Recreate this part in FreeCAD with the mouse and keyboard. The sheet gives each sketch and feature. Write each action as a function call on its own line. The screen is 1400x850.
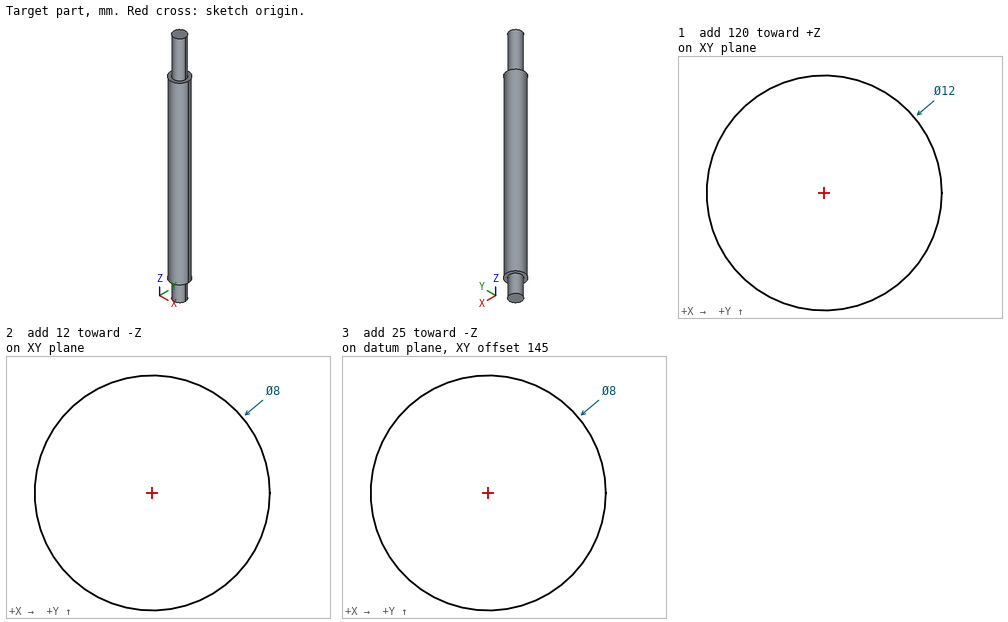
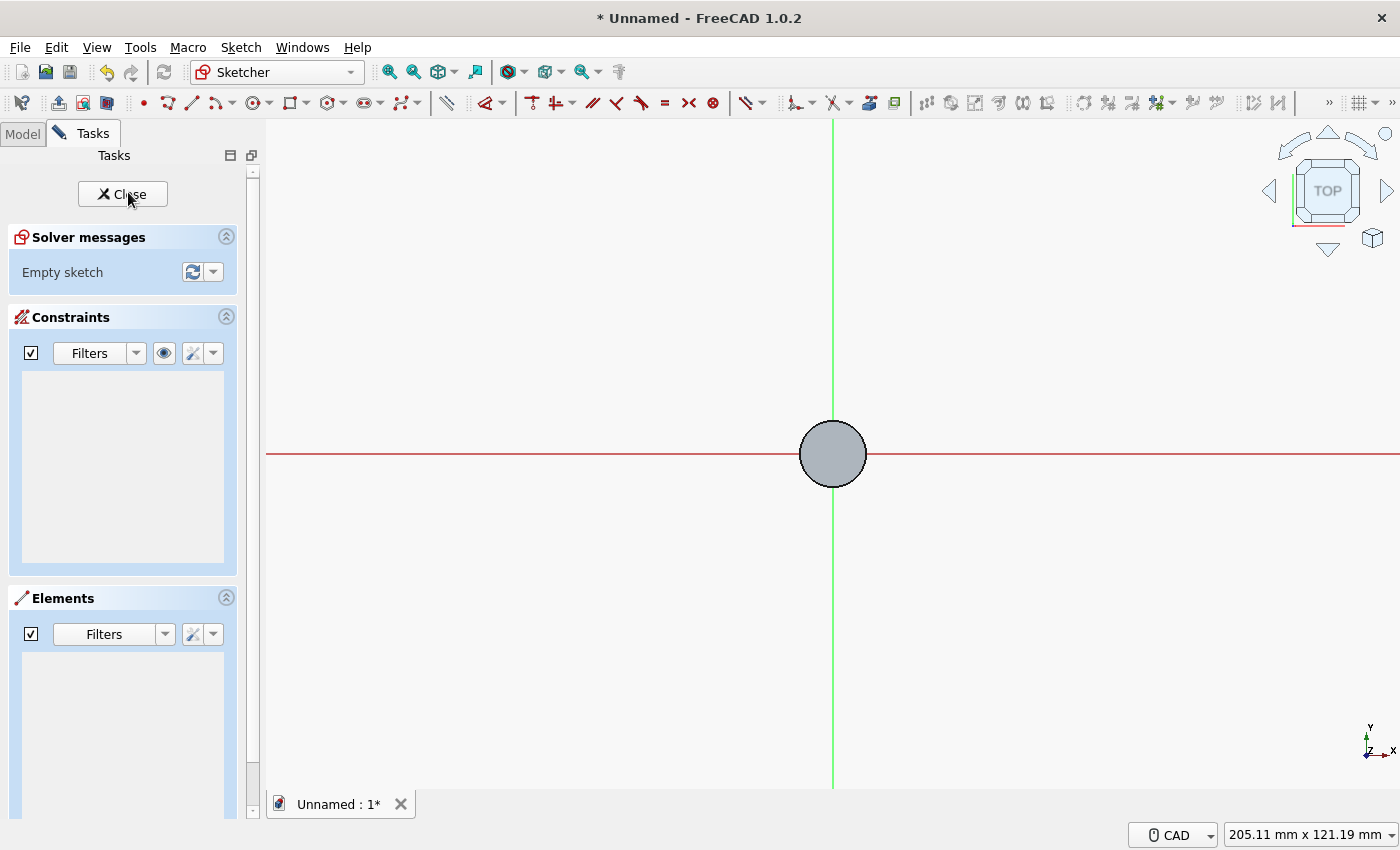
click(108, 104)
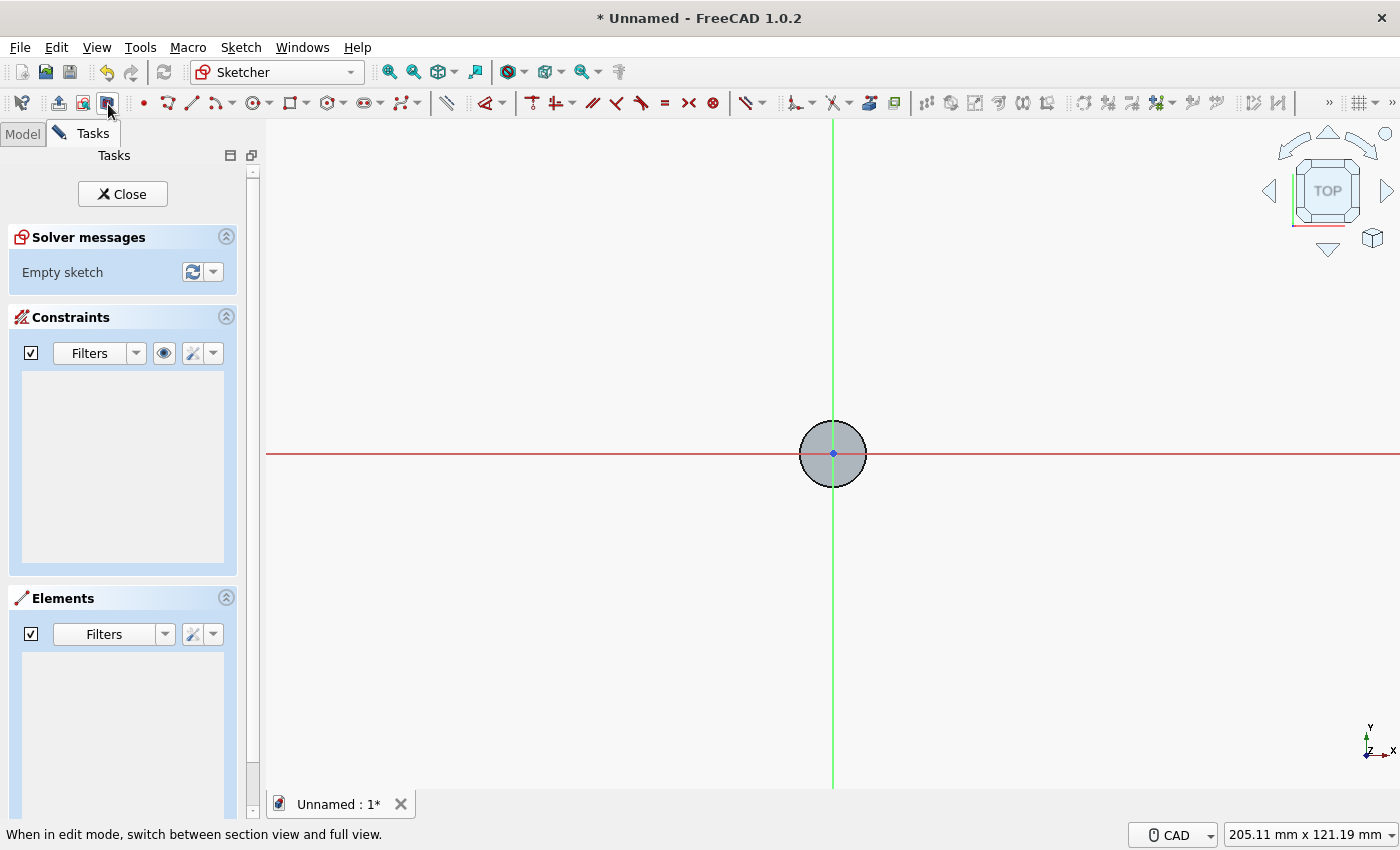
scroll(842, 454, up, 11)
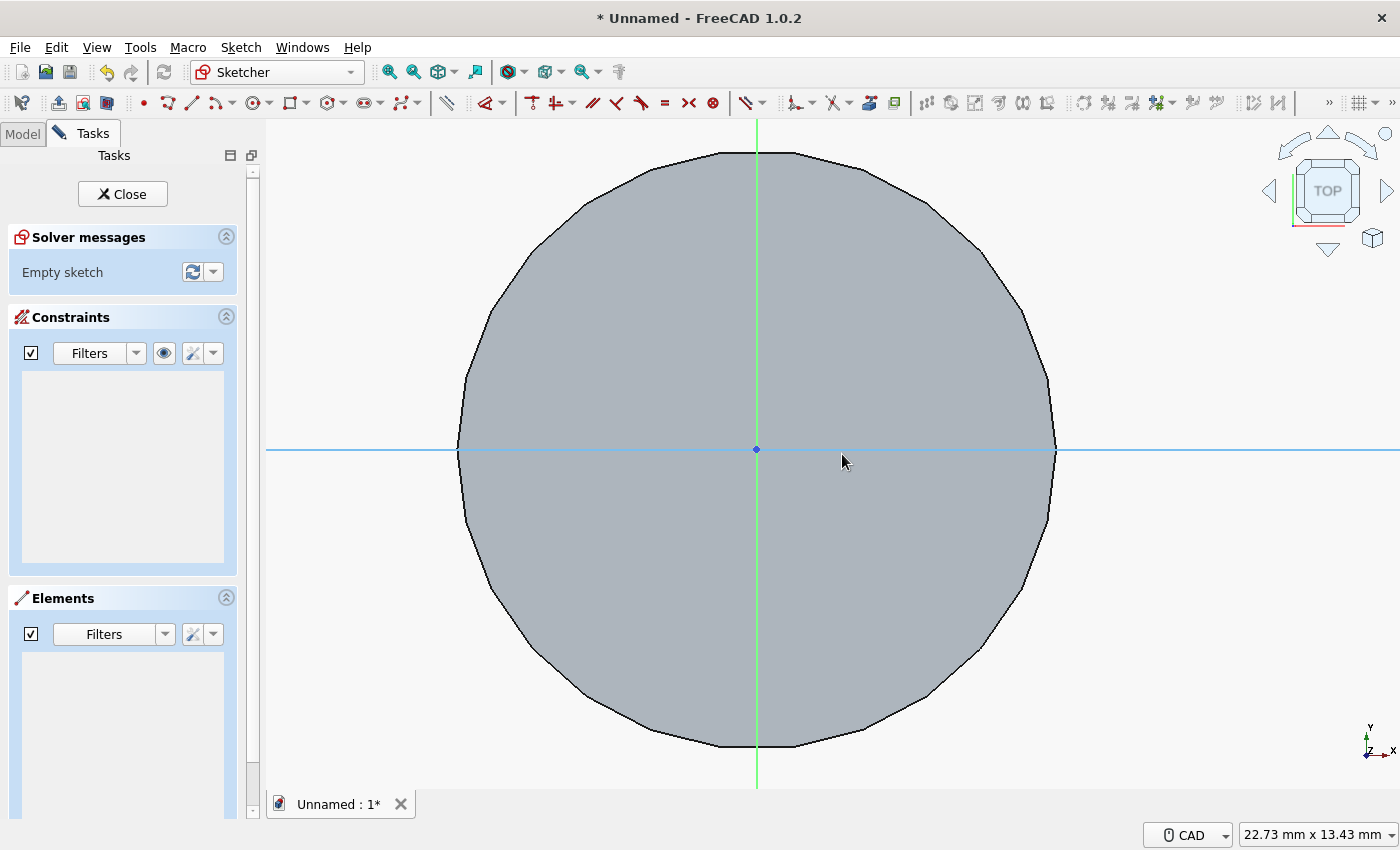
click(254, 104)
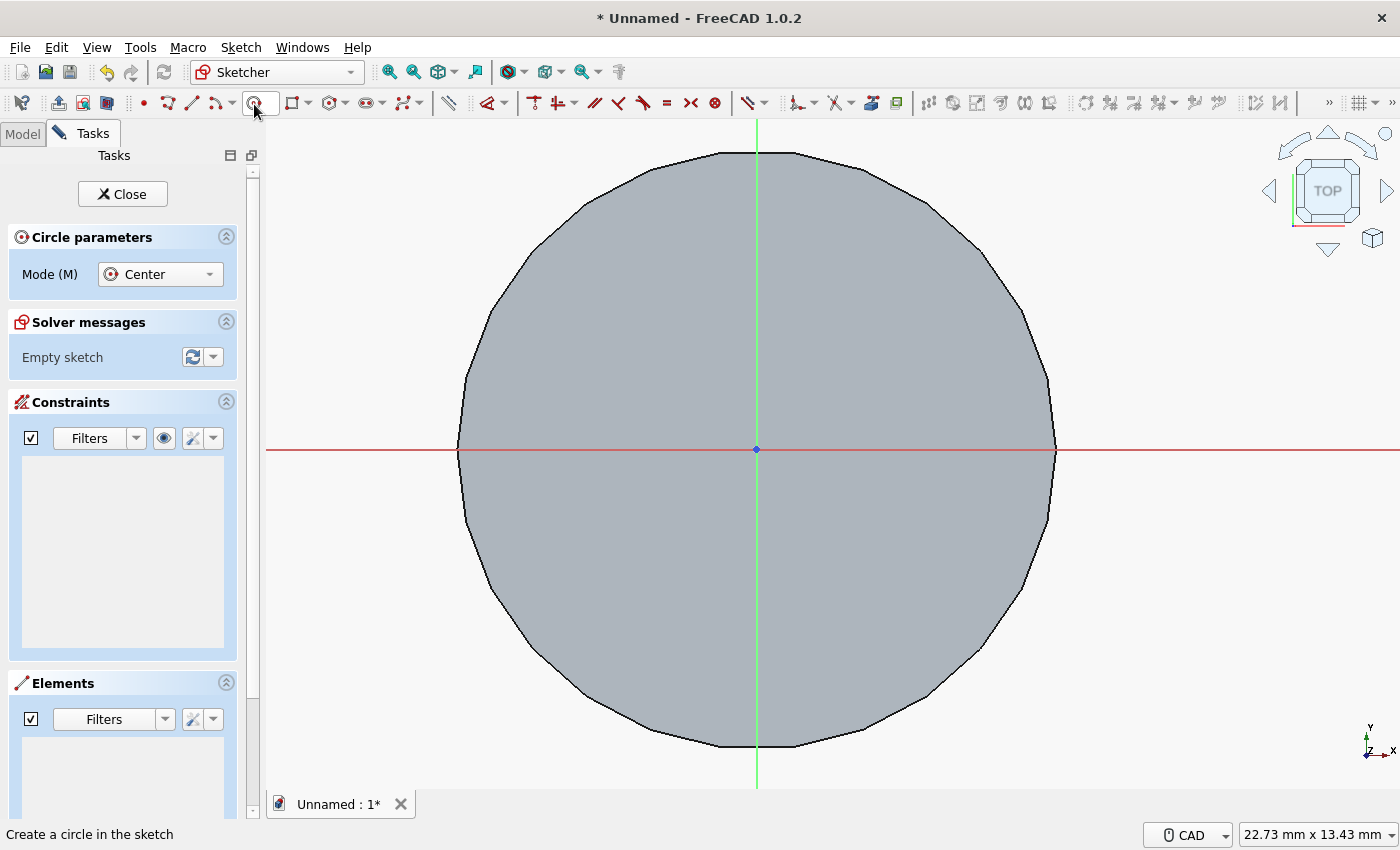
click(757, 450)
click(898, 309)
key(Escape)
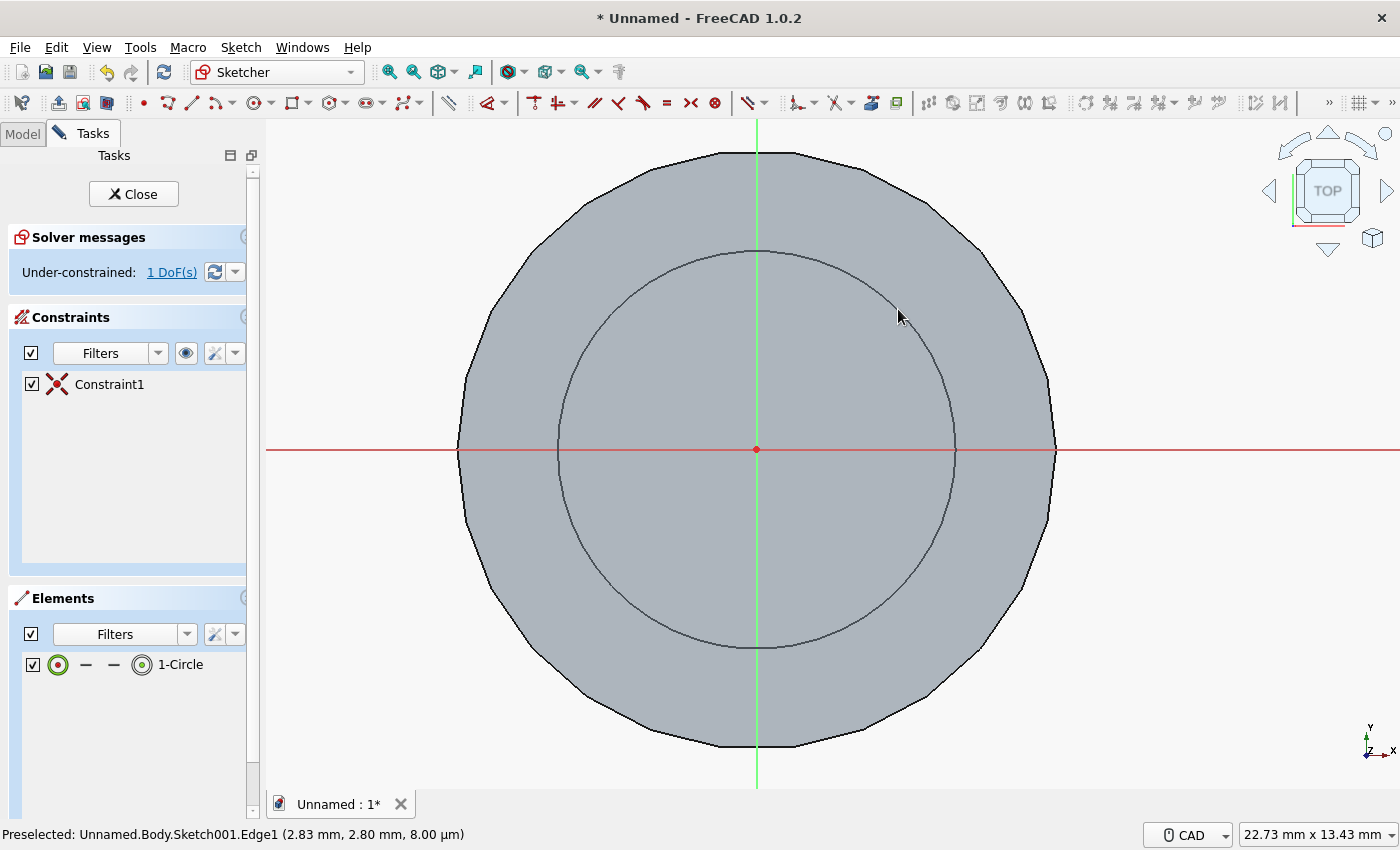
click(488, 104)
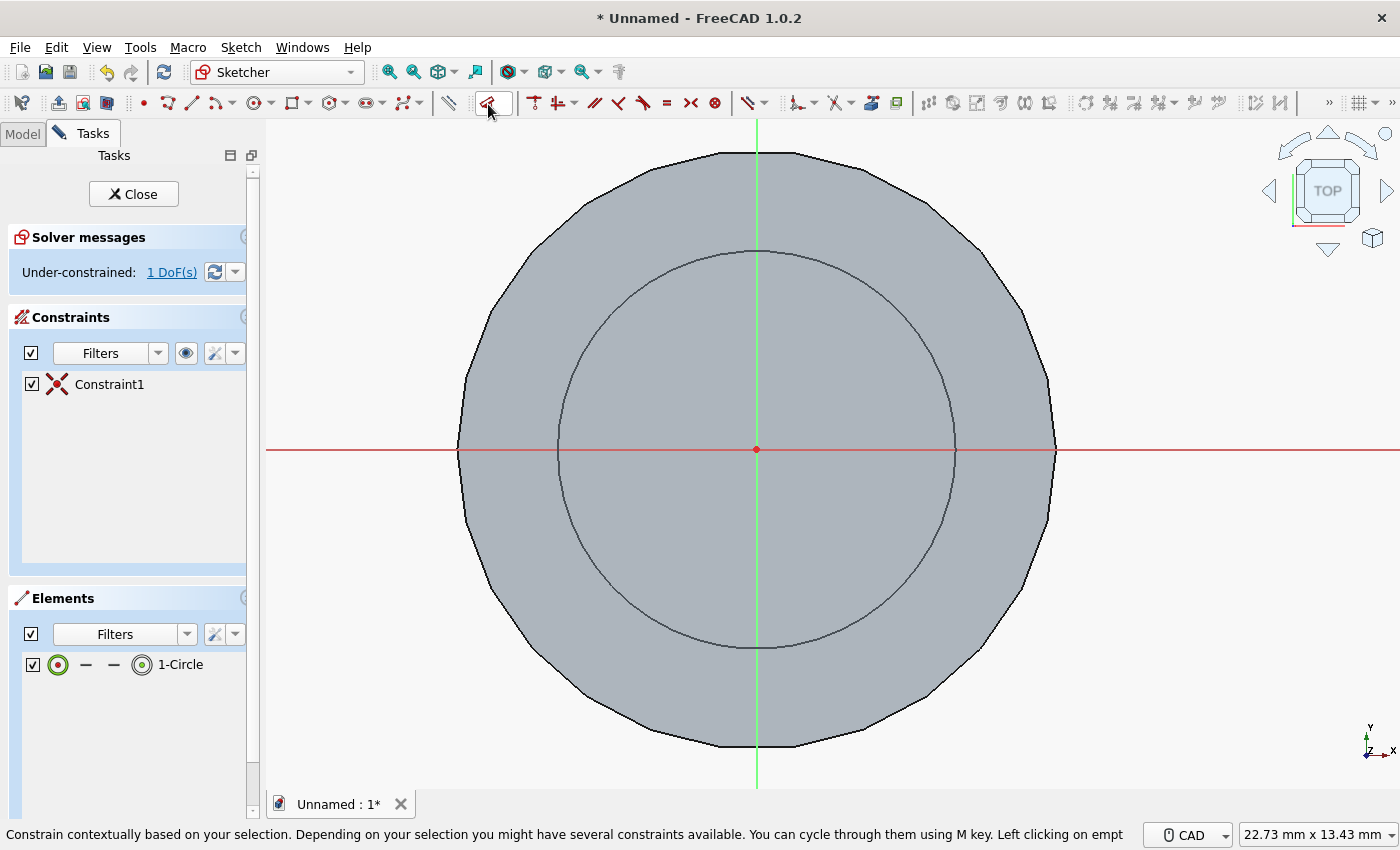
click(897, 309)
click(920, 286)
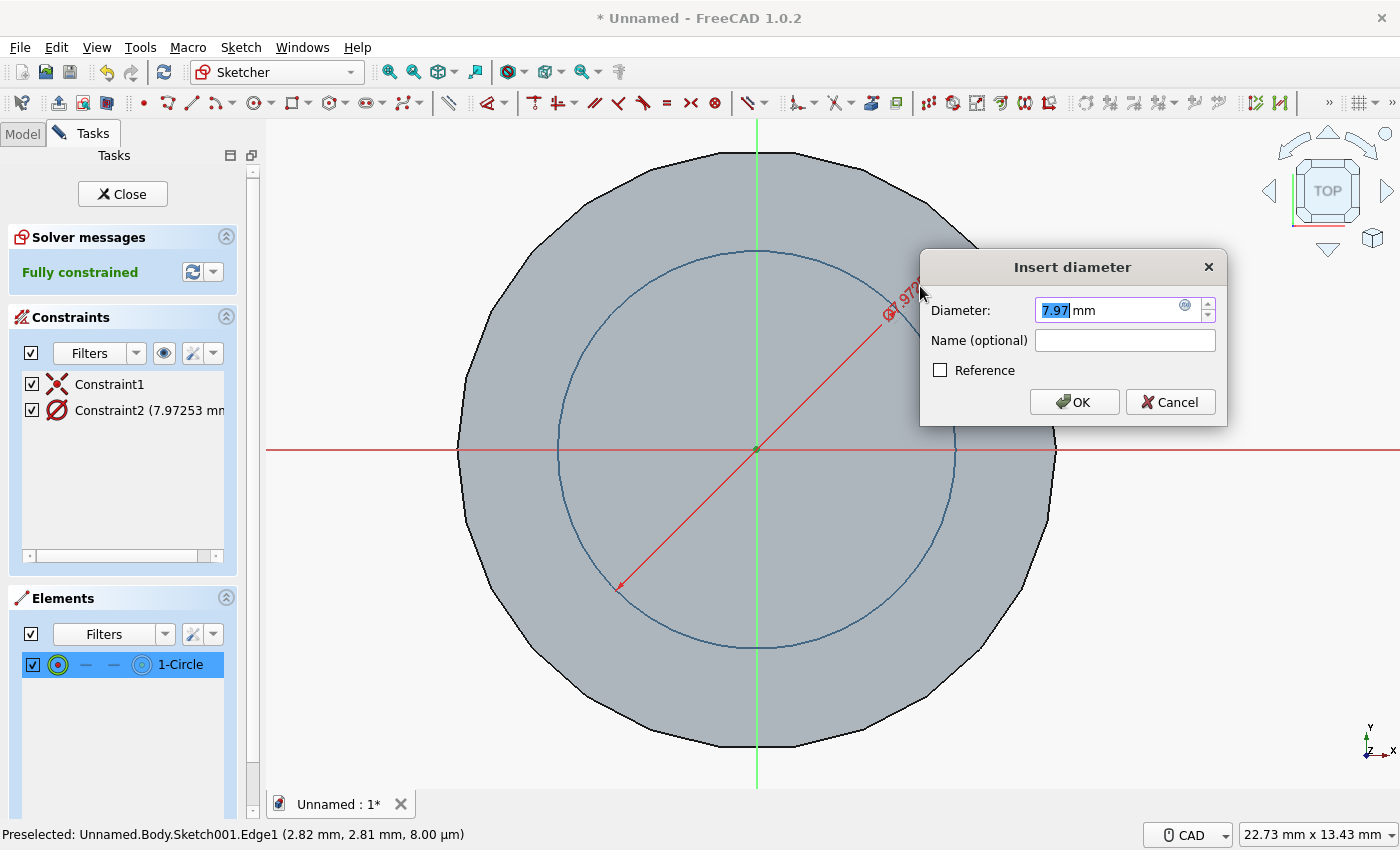
text(8)
key(Return)
key(Escape)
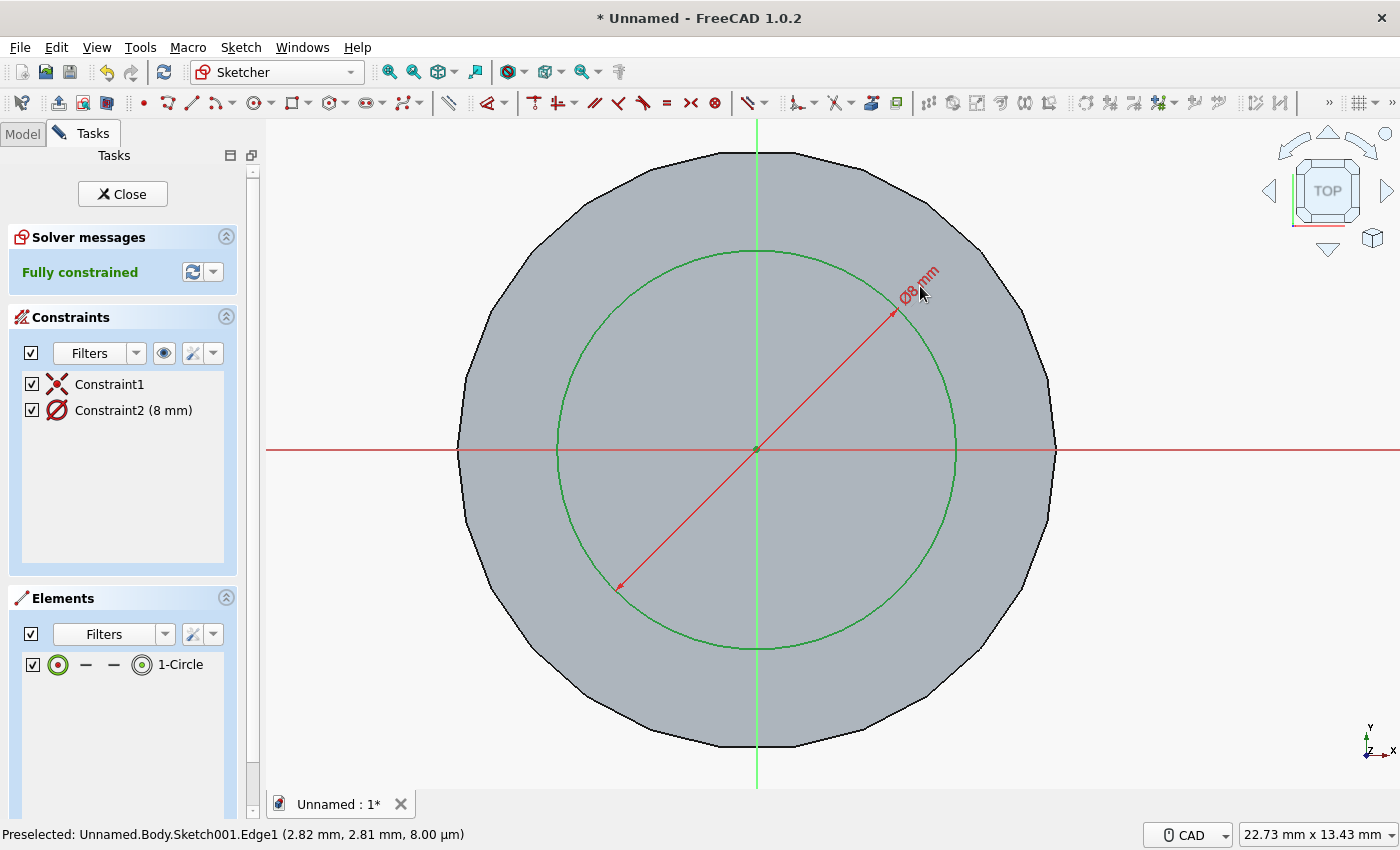
click(123, 194)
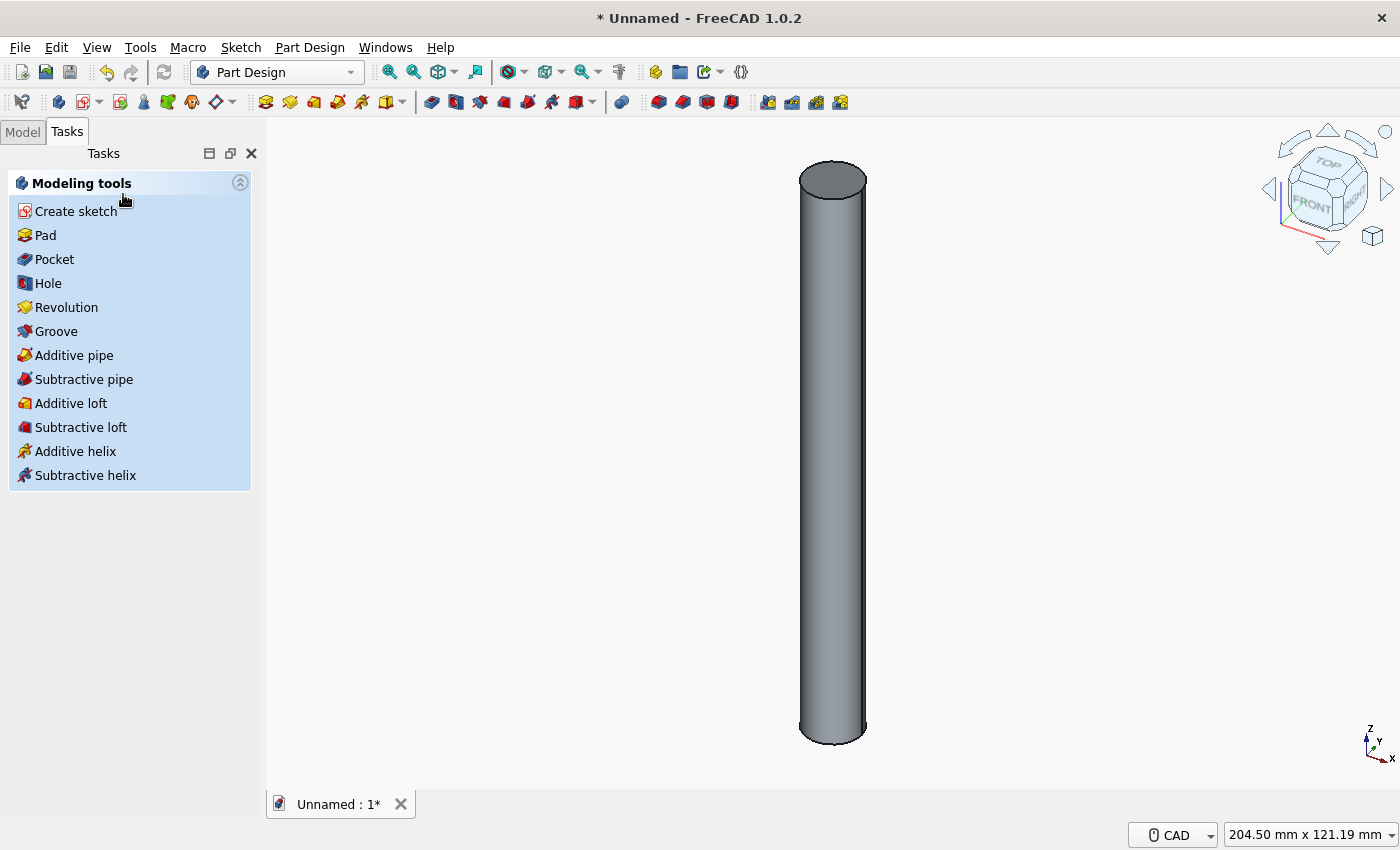
click(266, 102)